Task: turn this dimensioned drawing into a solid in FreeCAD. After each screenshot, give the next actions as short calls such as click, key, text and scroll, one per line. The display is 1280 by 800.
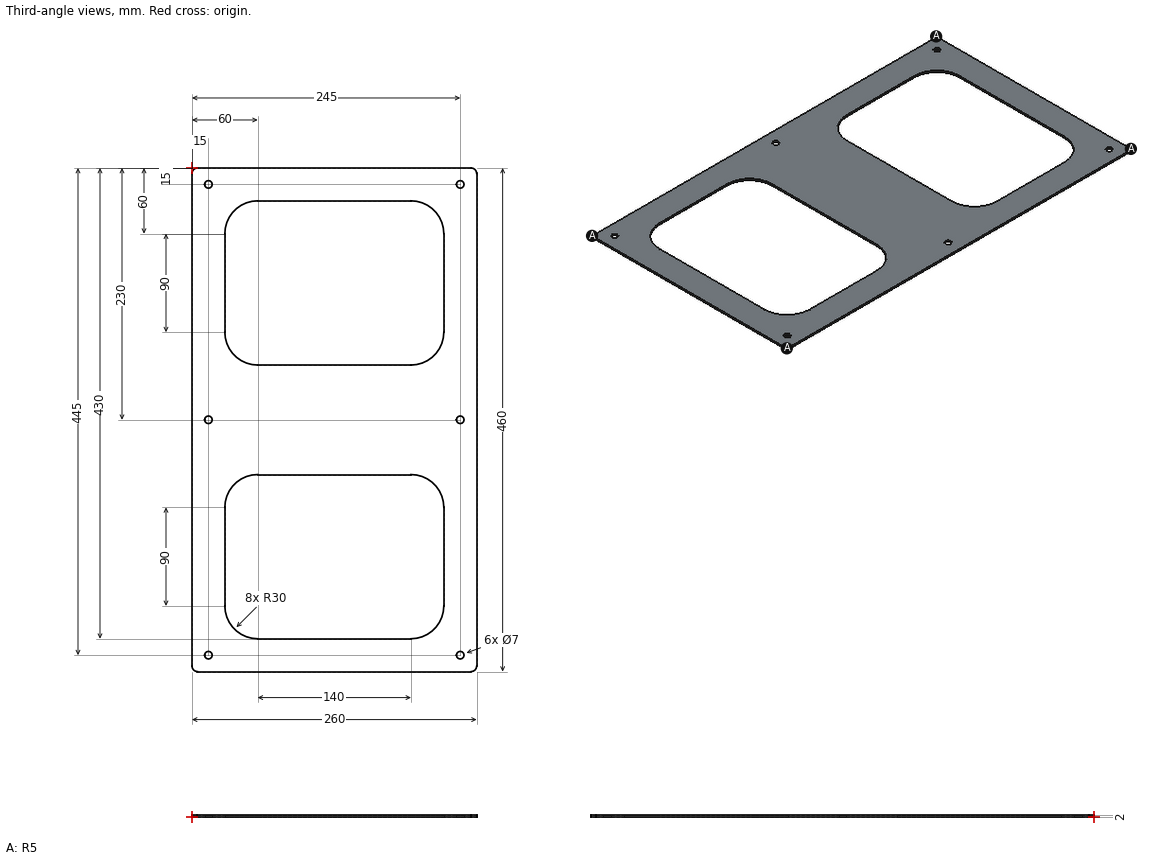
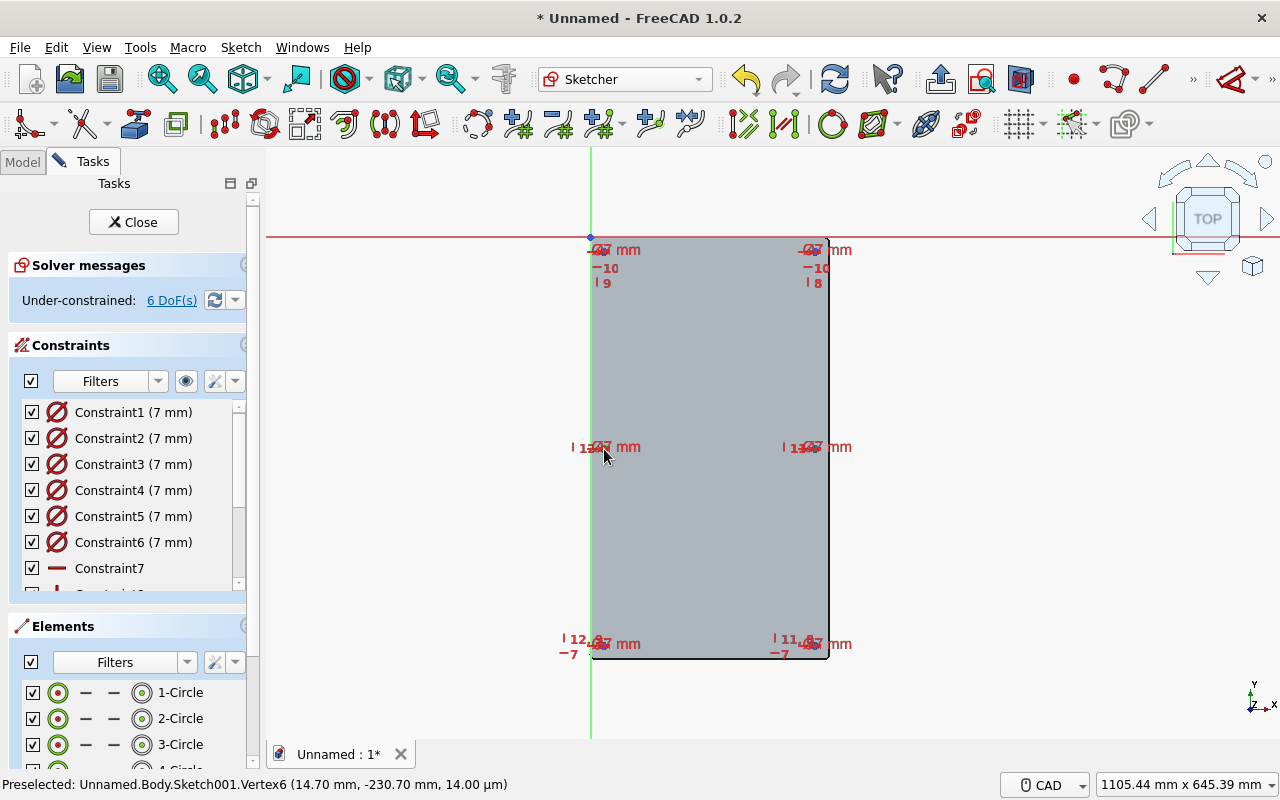
key(h)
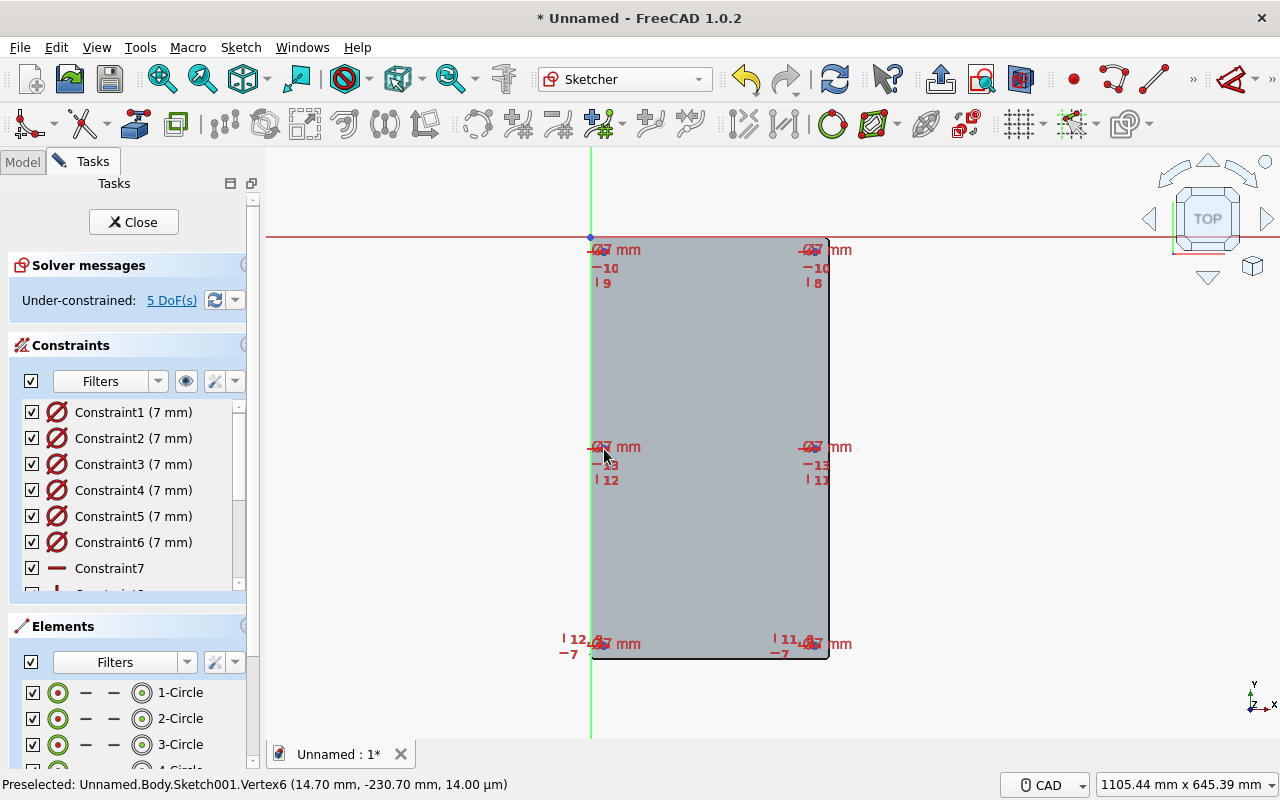
click(1232, 80)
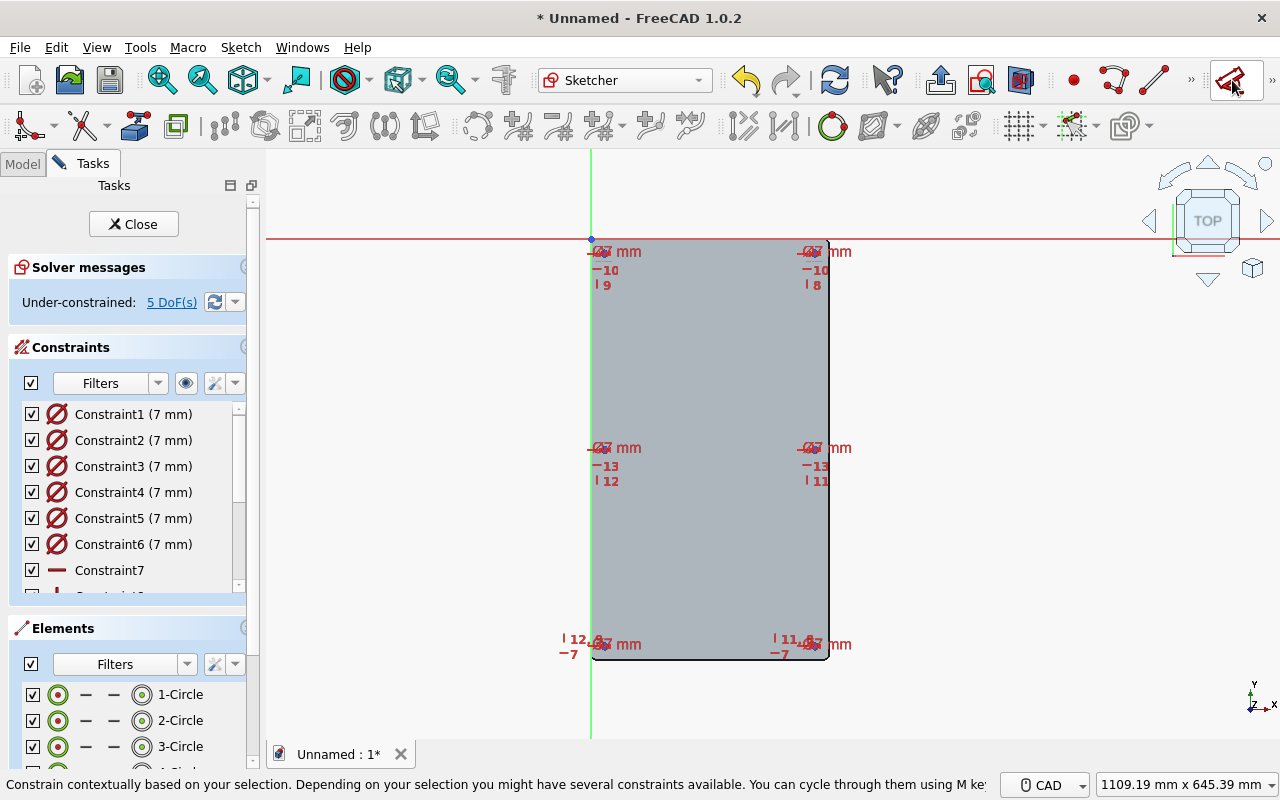
scroll(605, 646, up, 6)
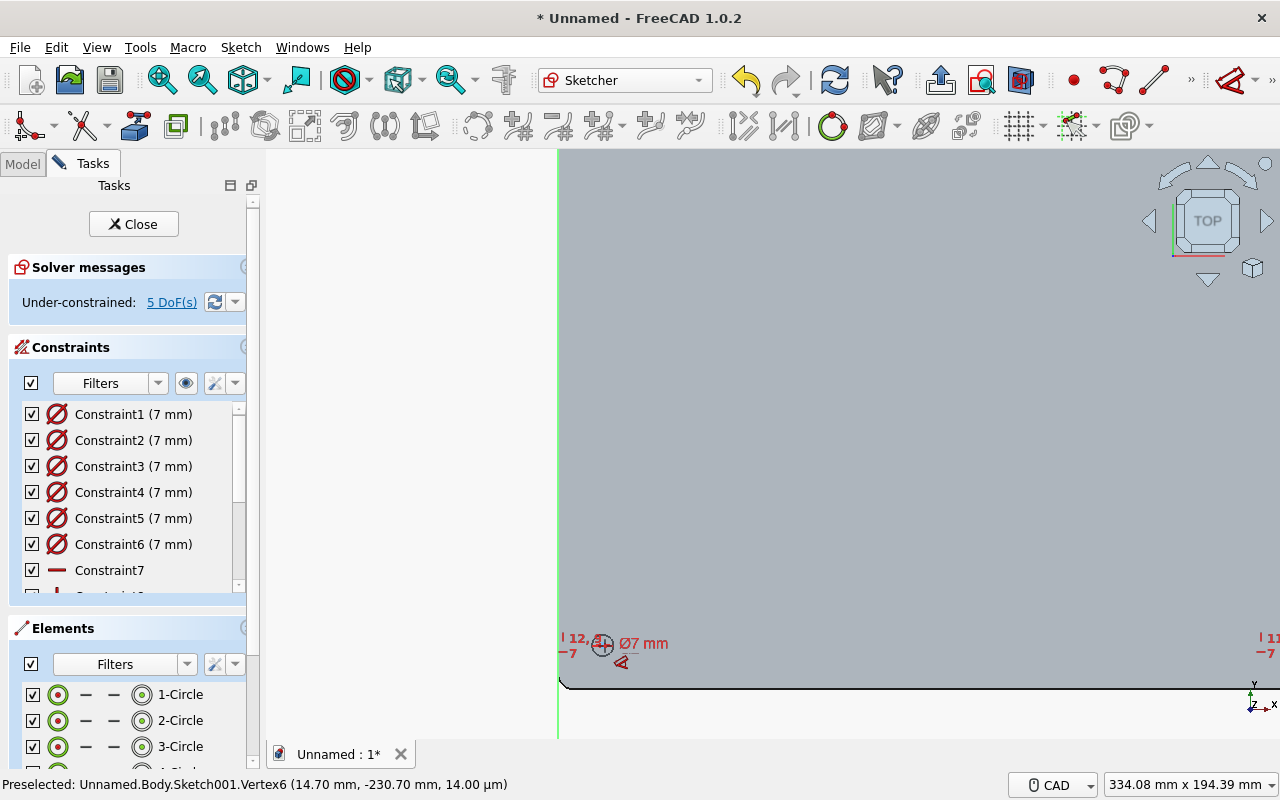
click(603, 646)
click(580, 680)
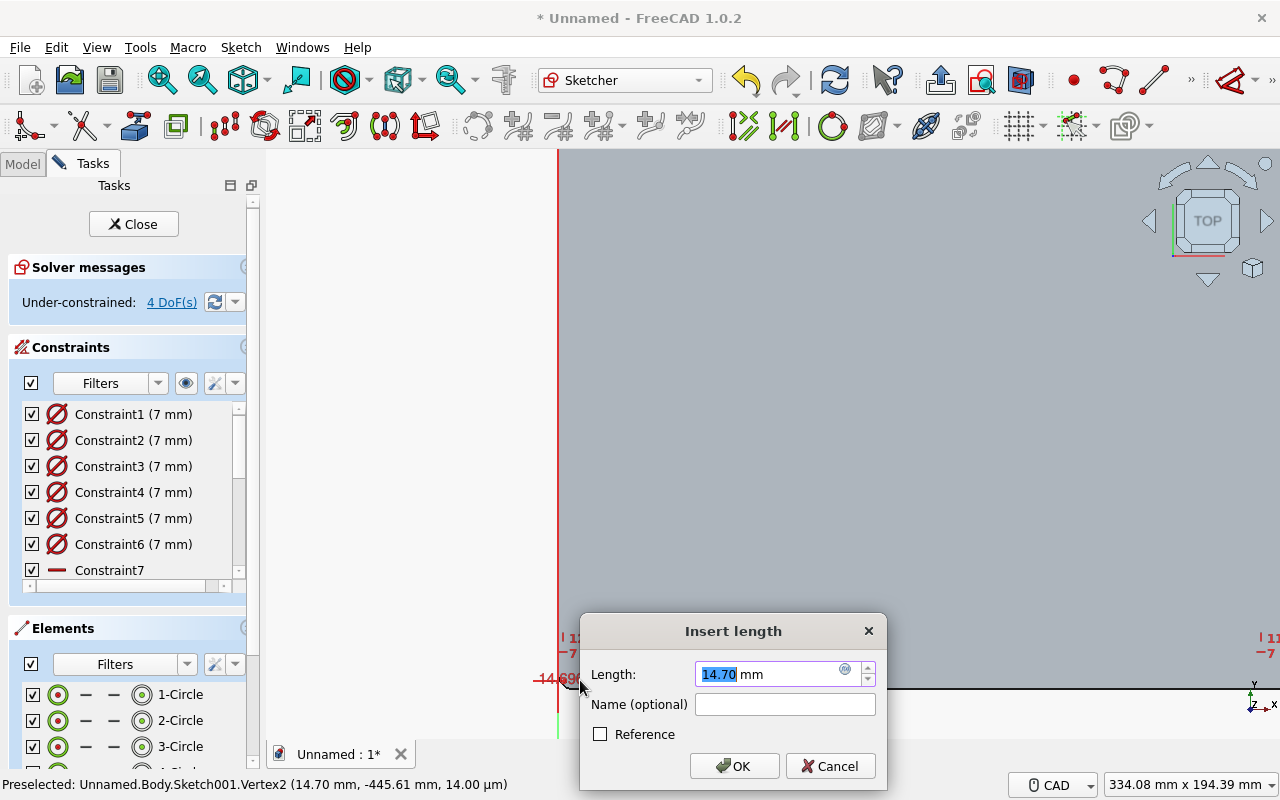
text(15)
key(Return)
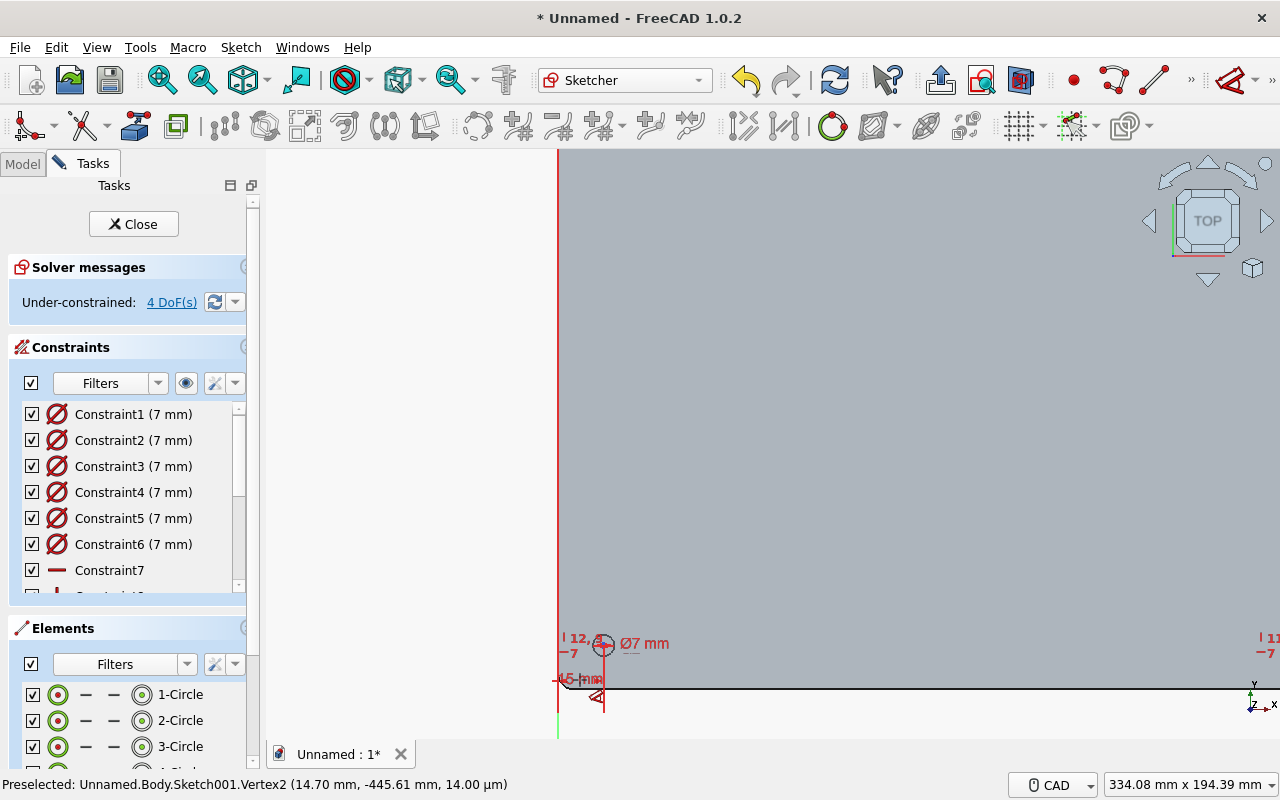
scroll(605, 647, down, 6)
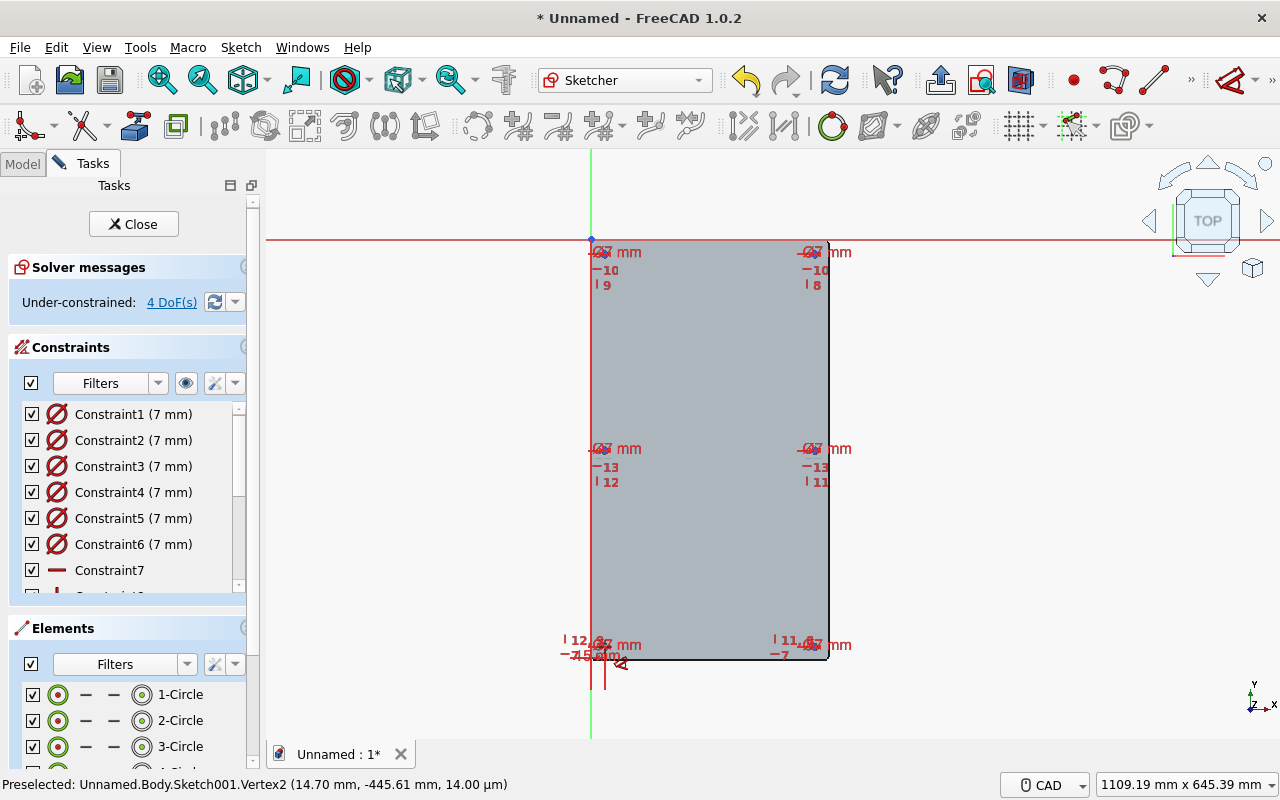
scroll(815, 254, up, 6)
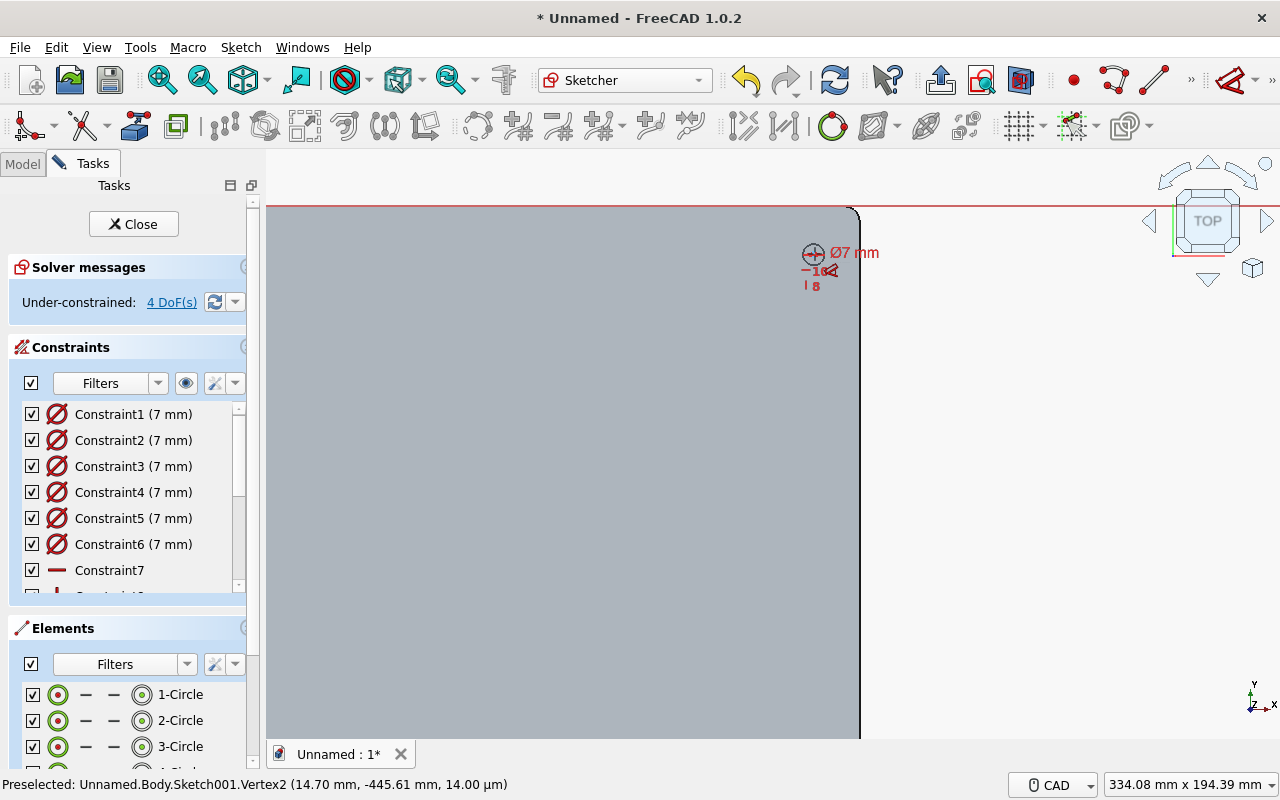
click(814, 255)
click(848, 231)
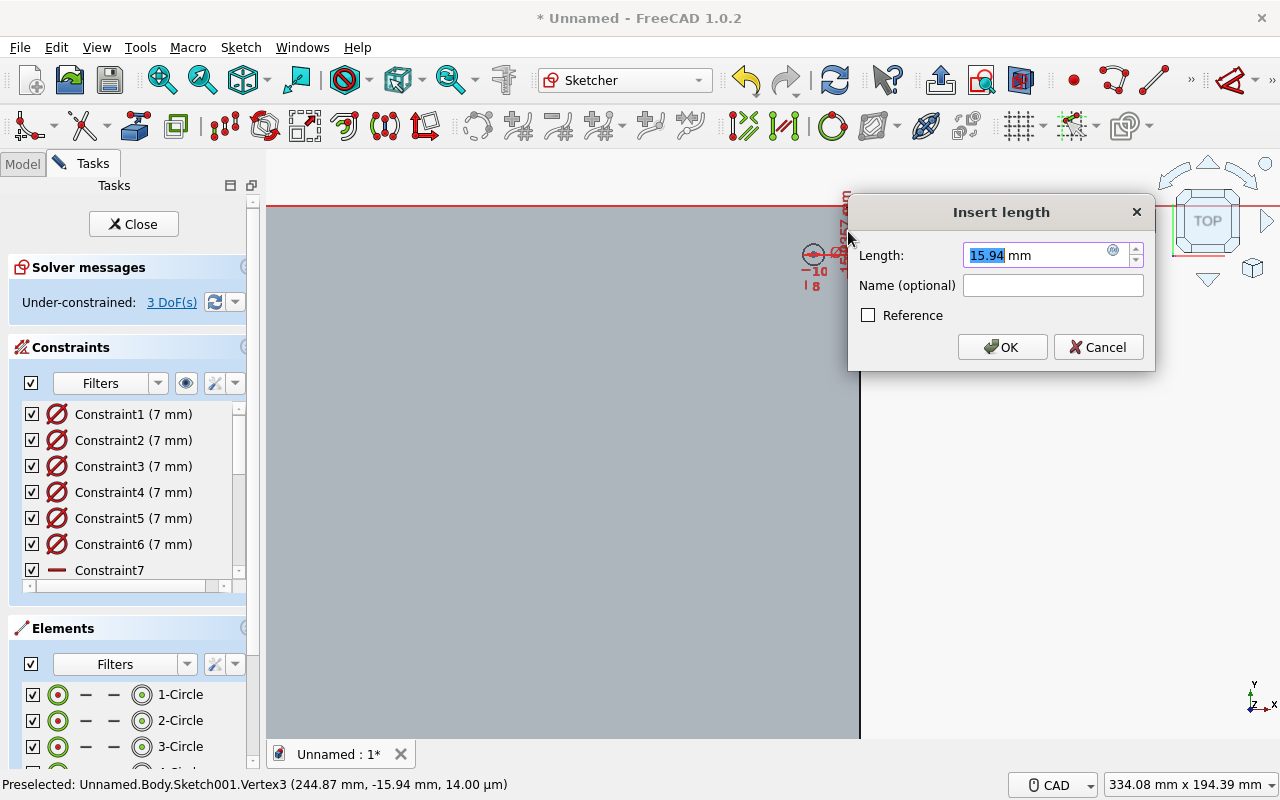
text(15)
key(Return)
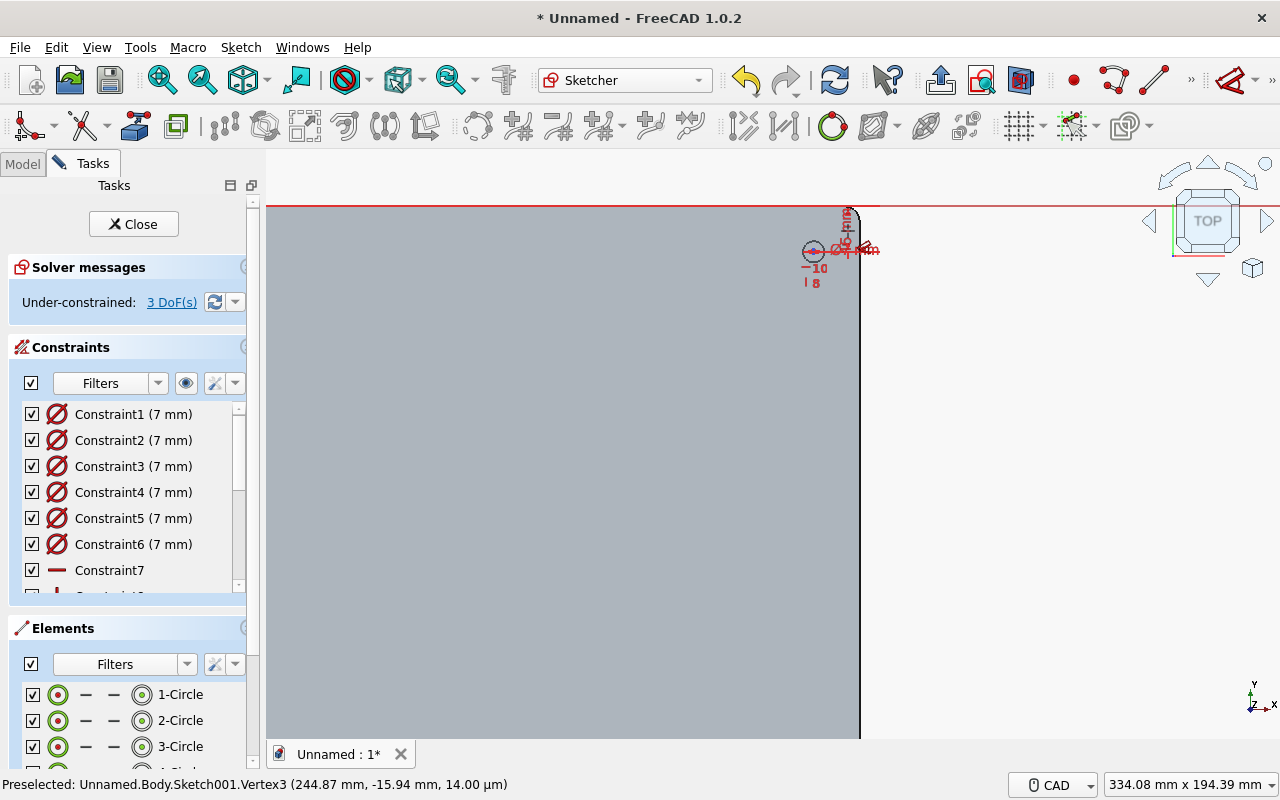
scroll(815, 253, down, 6)